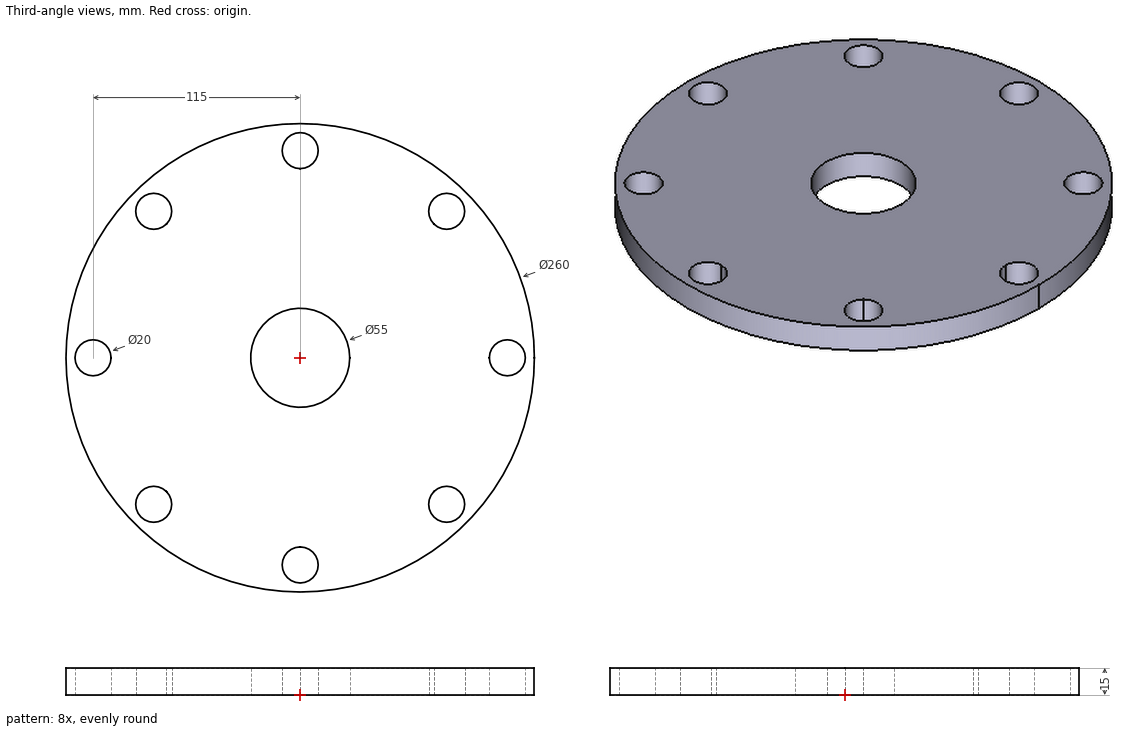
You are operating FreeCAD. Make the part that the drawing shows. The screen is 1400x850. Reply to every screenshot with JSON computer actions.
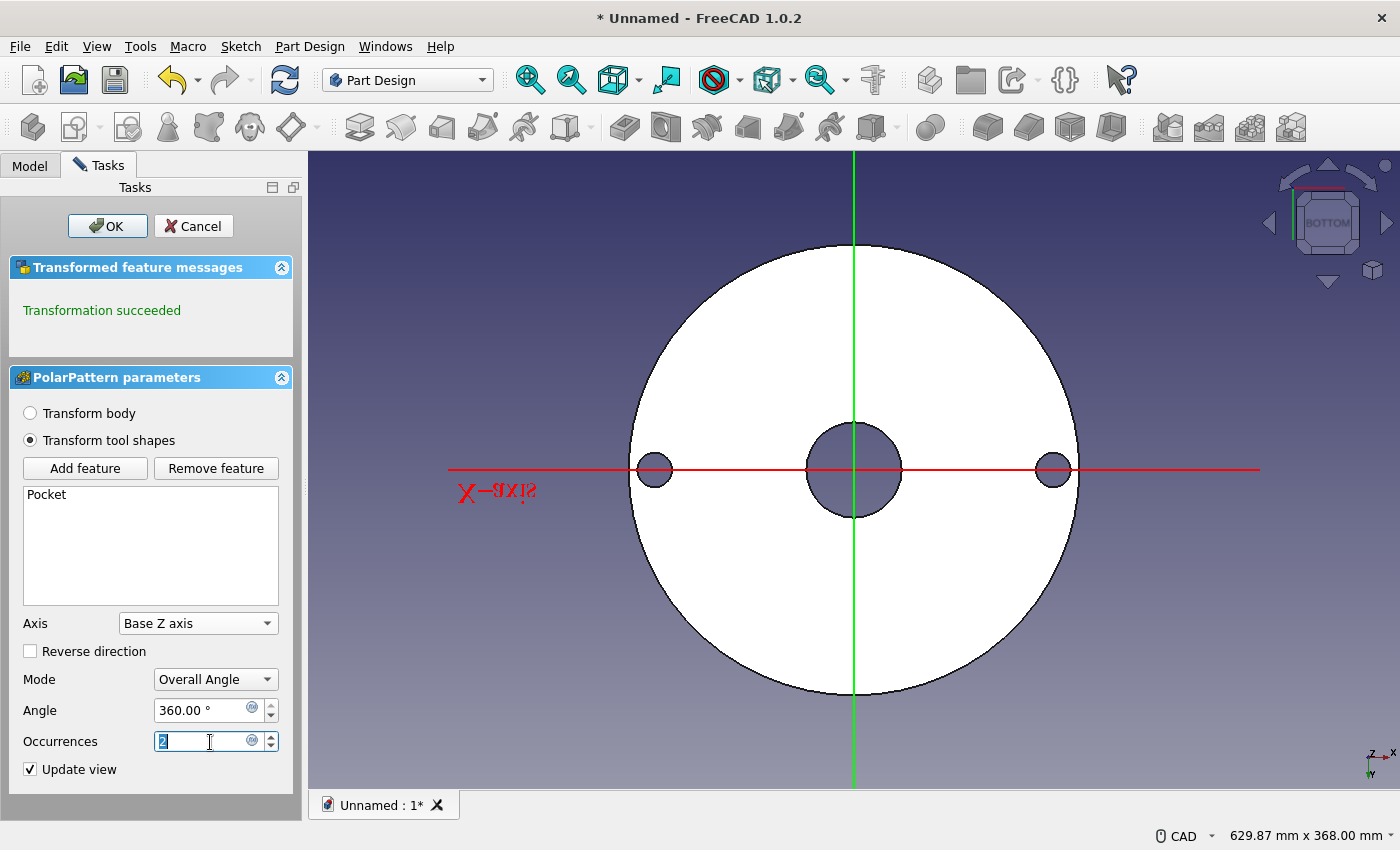
{"action": "type", "text": "8"}
{"action": "key", "text": "Tab"}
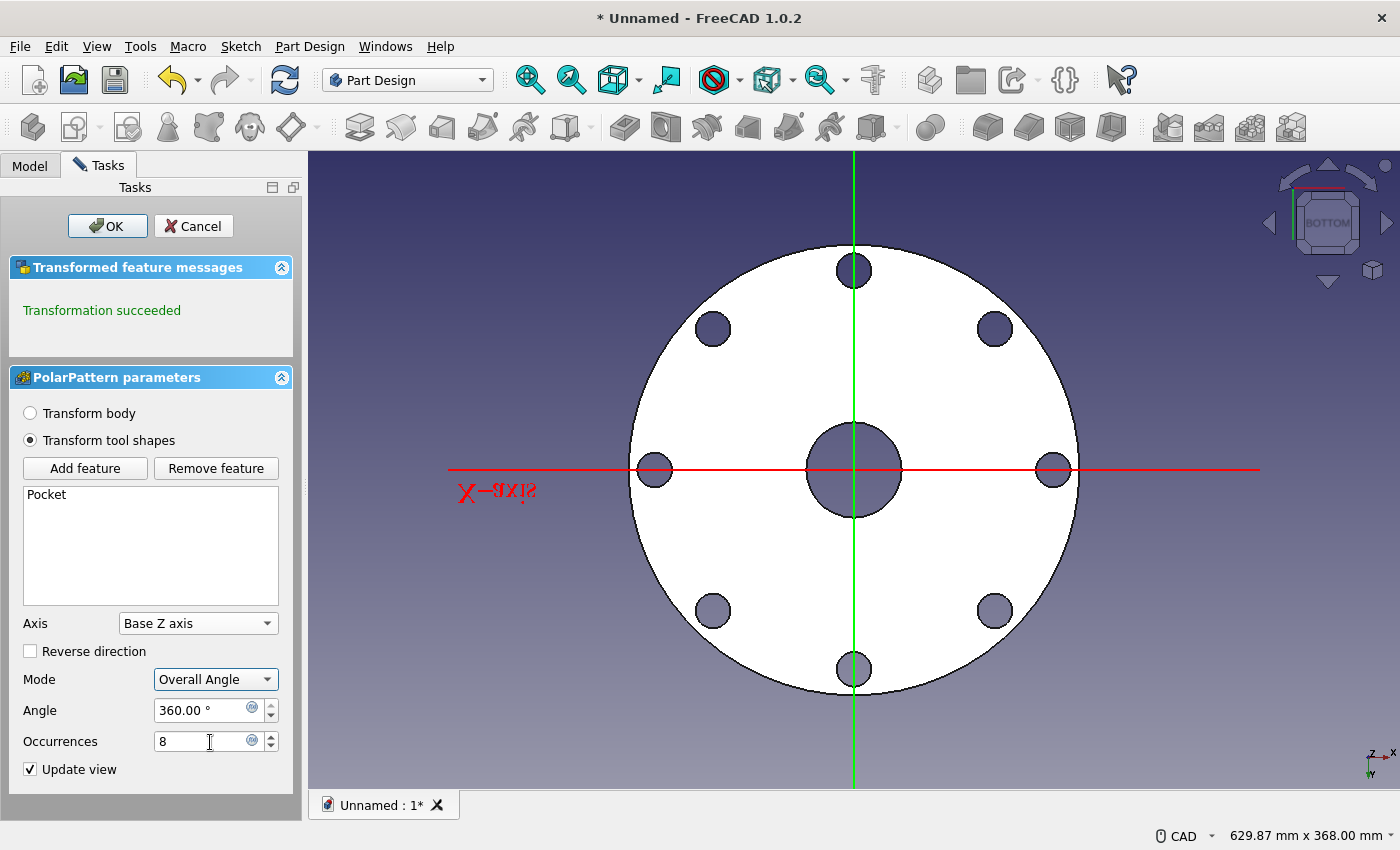
{"action": "left_click", "coordinate": [108, 226]}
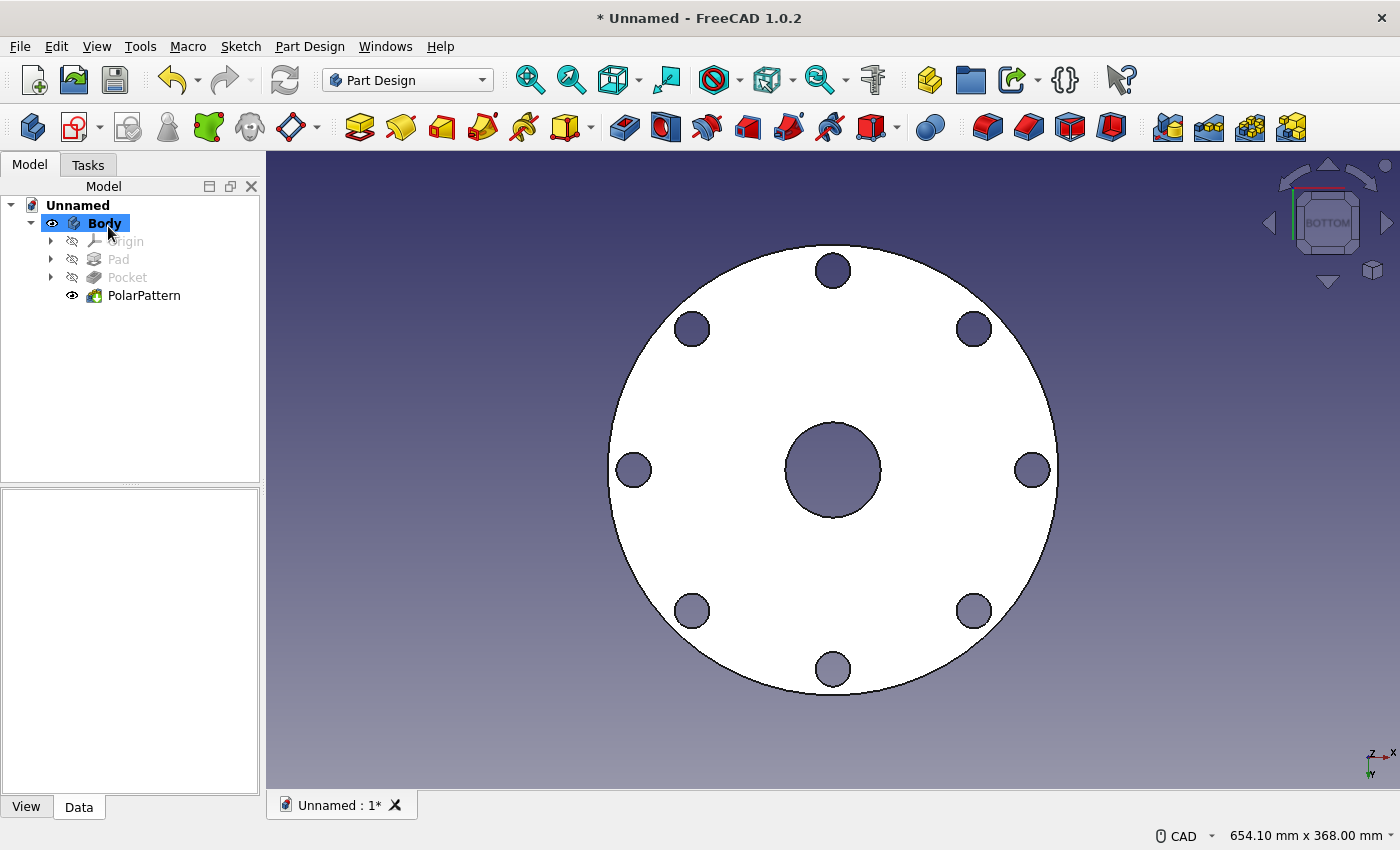
{"action": "key", "text": "0"}